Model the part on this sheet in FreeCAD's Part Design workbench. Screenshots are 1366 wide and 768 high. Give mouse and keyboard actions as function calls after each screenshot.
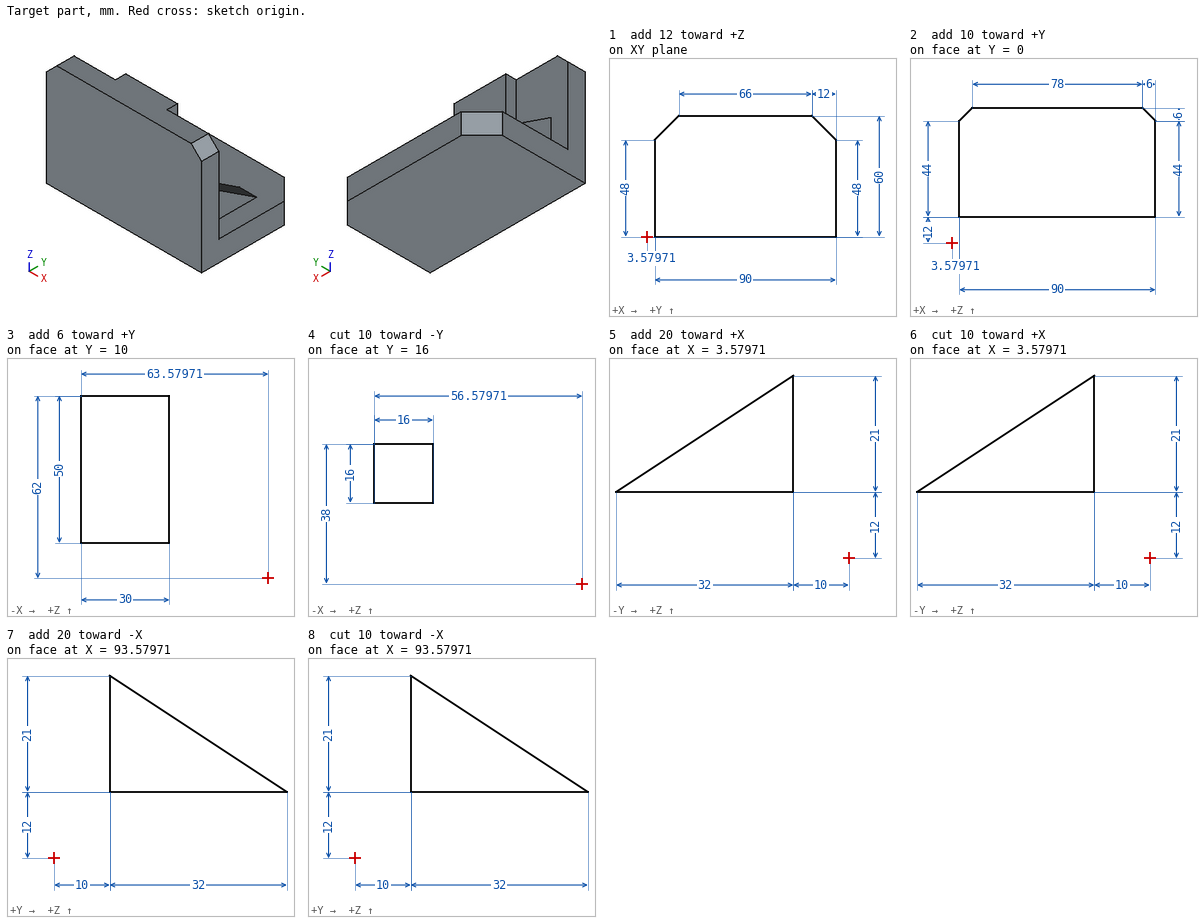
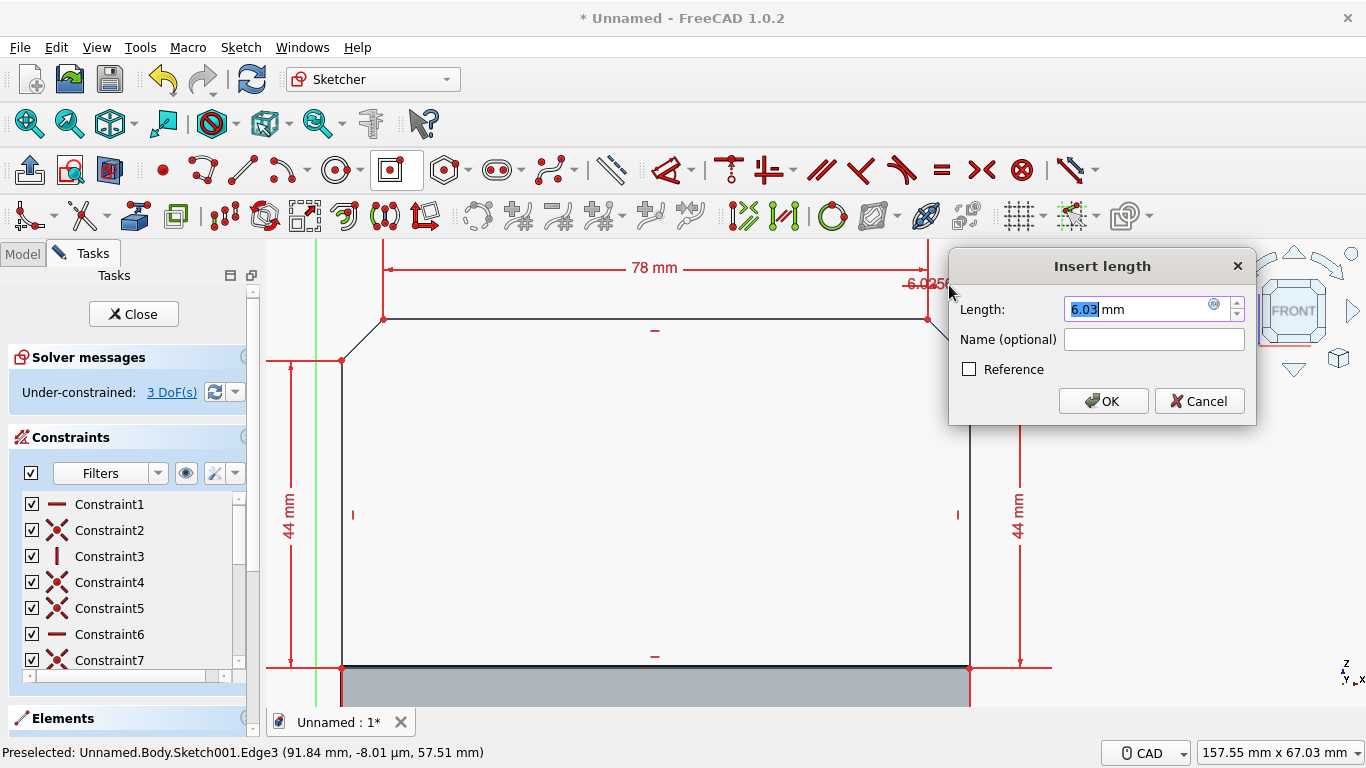
text(6)
key(Return)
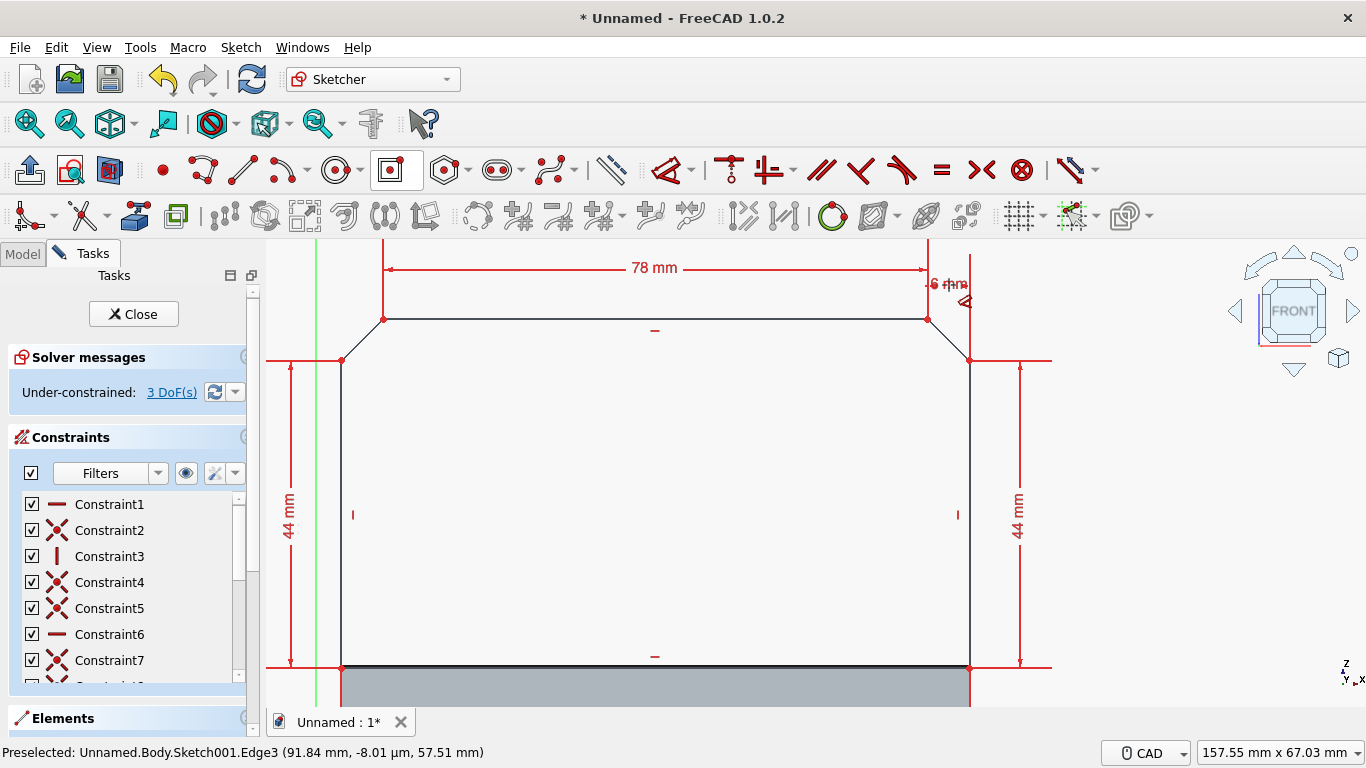
click(957, 348)
click(1004, 340)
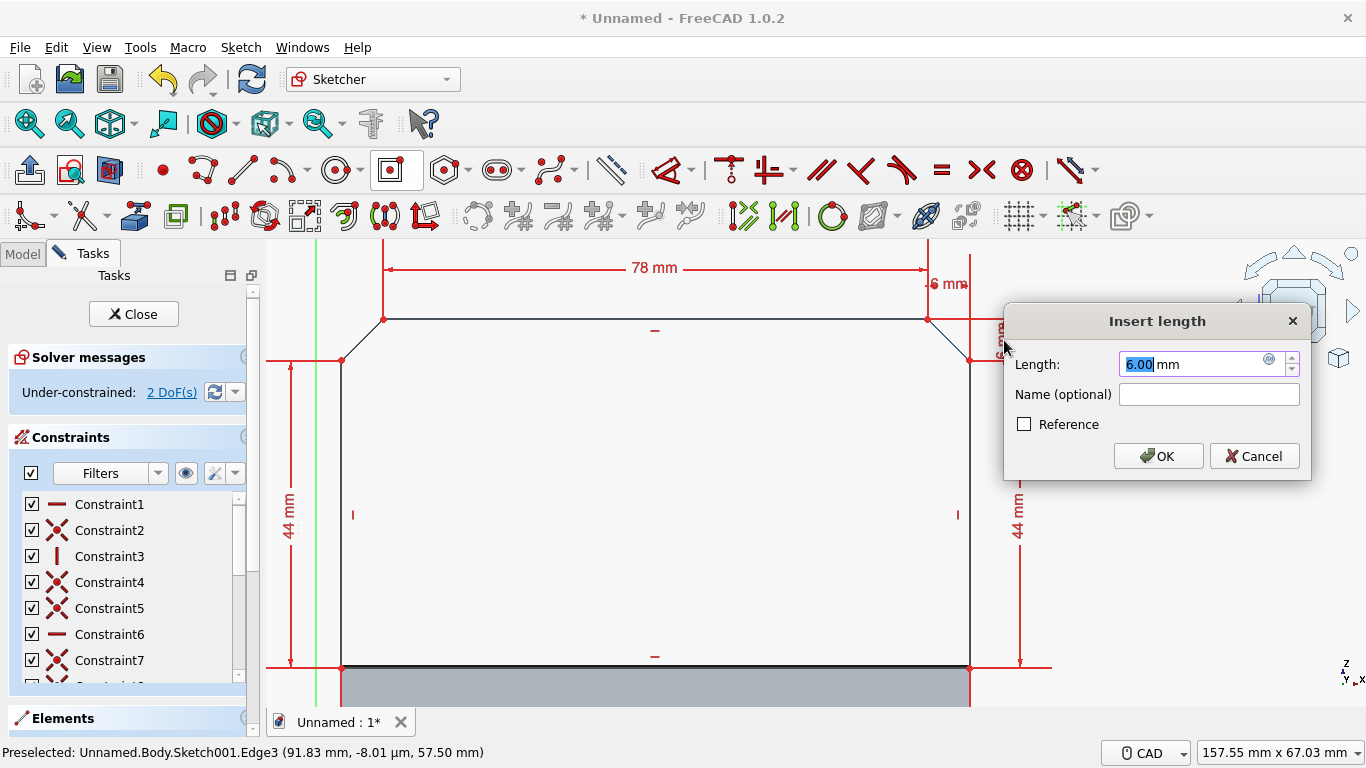
text(6)
key(Return)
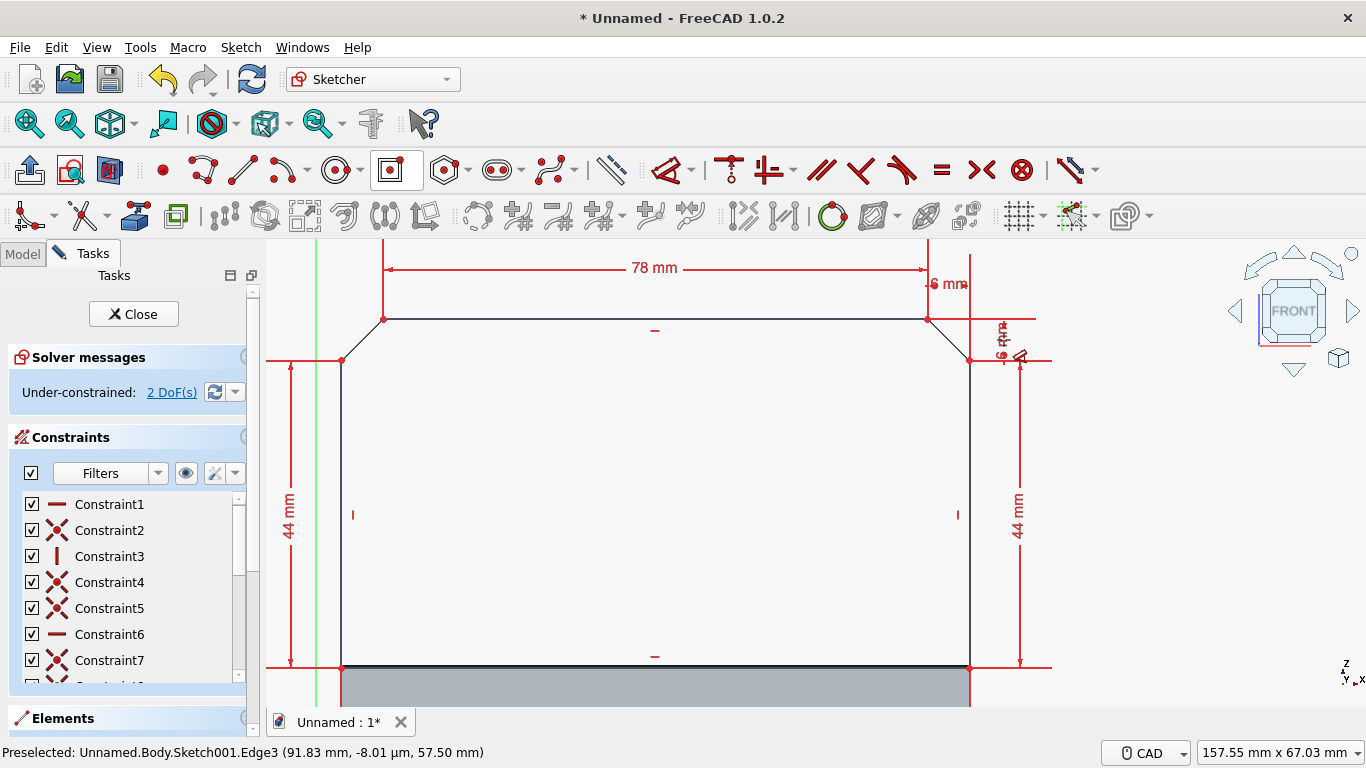
click(341, 668)
click(375, 676)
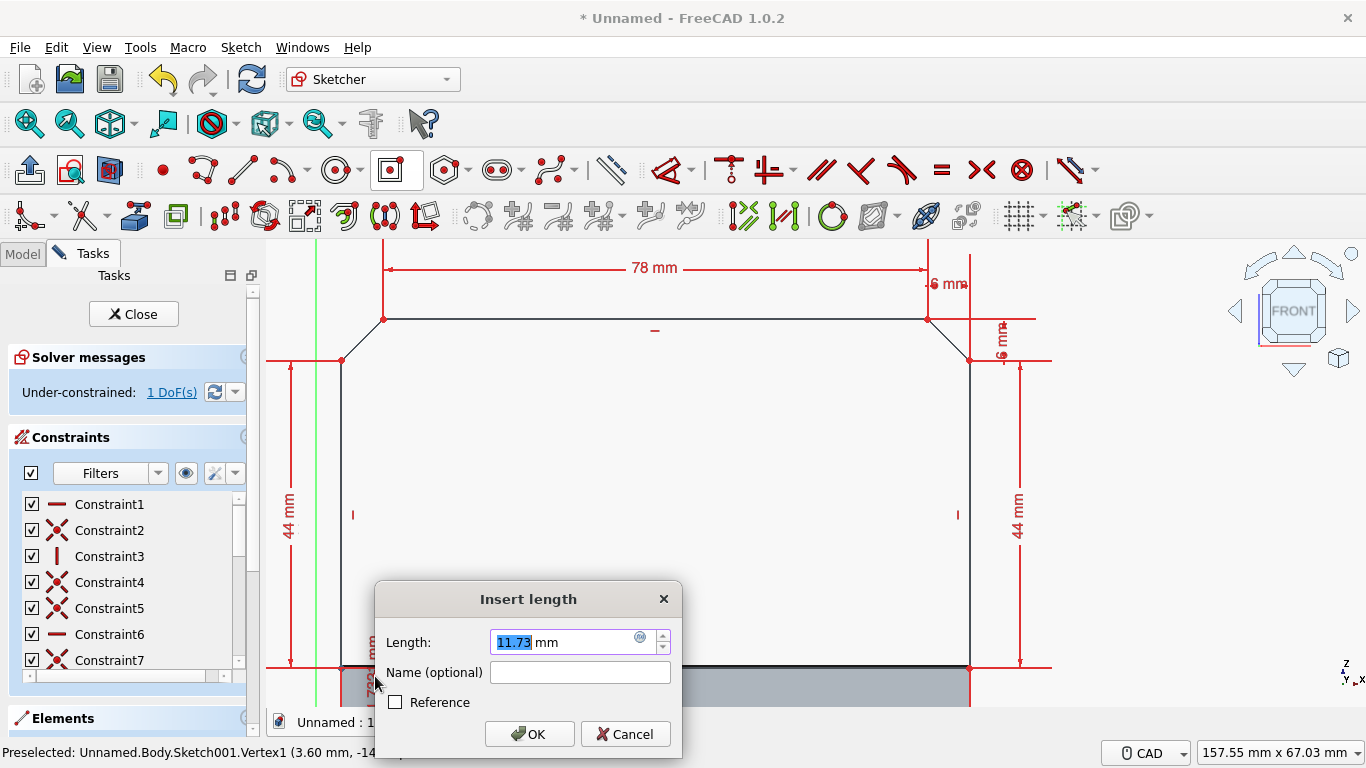
text(12)
key(Return)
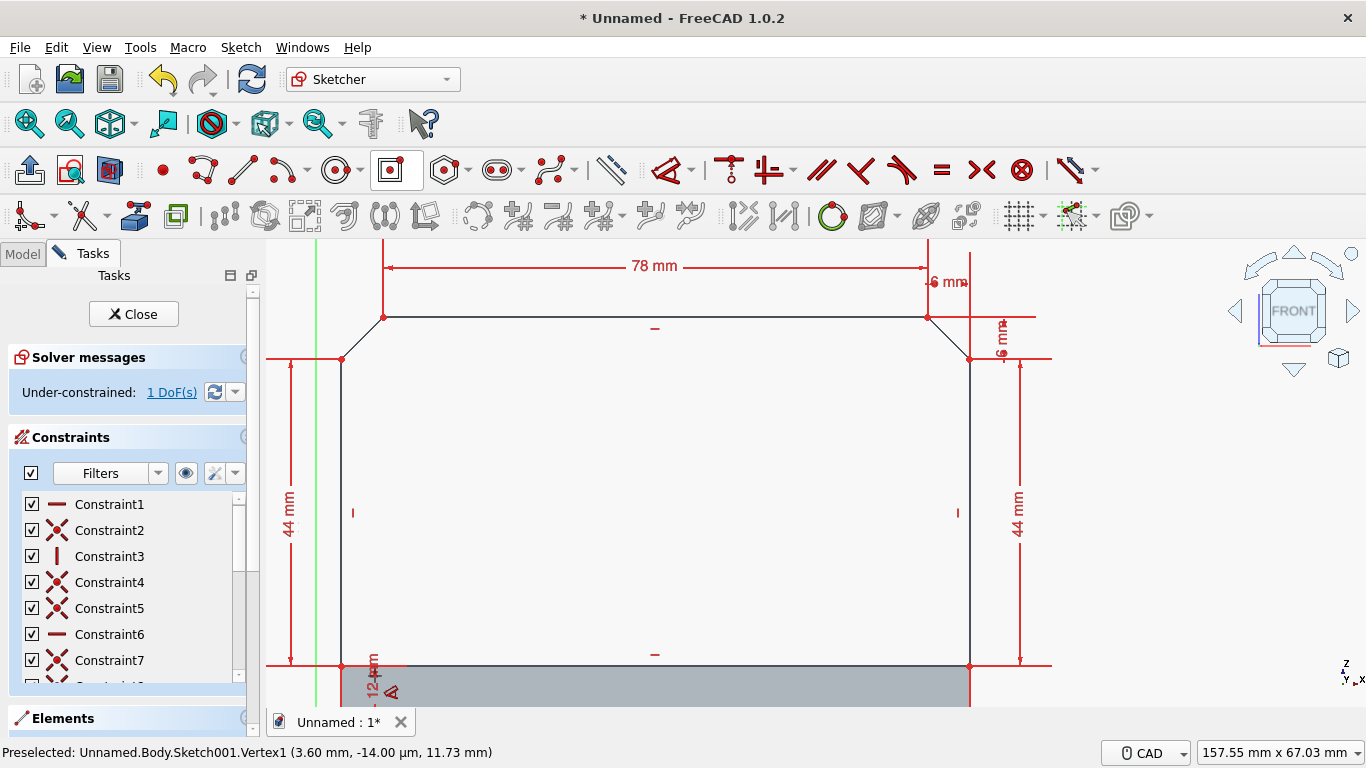
scroll(341, 666, up, 3)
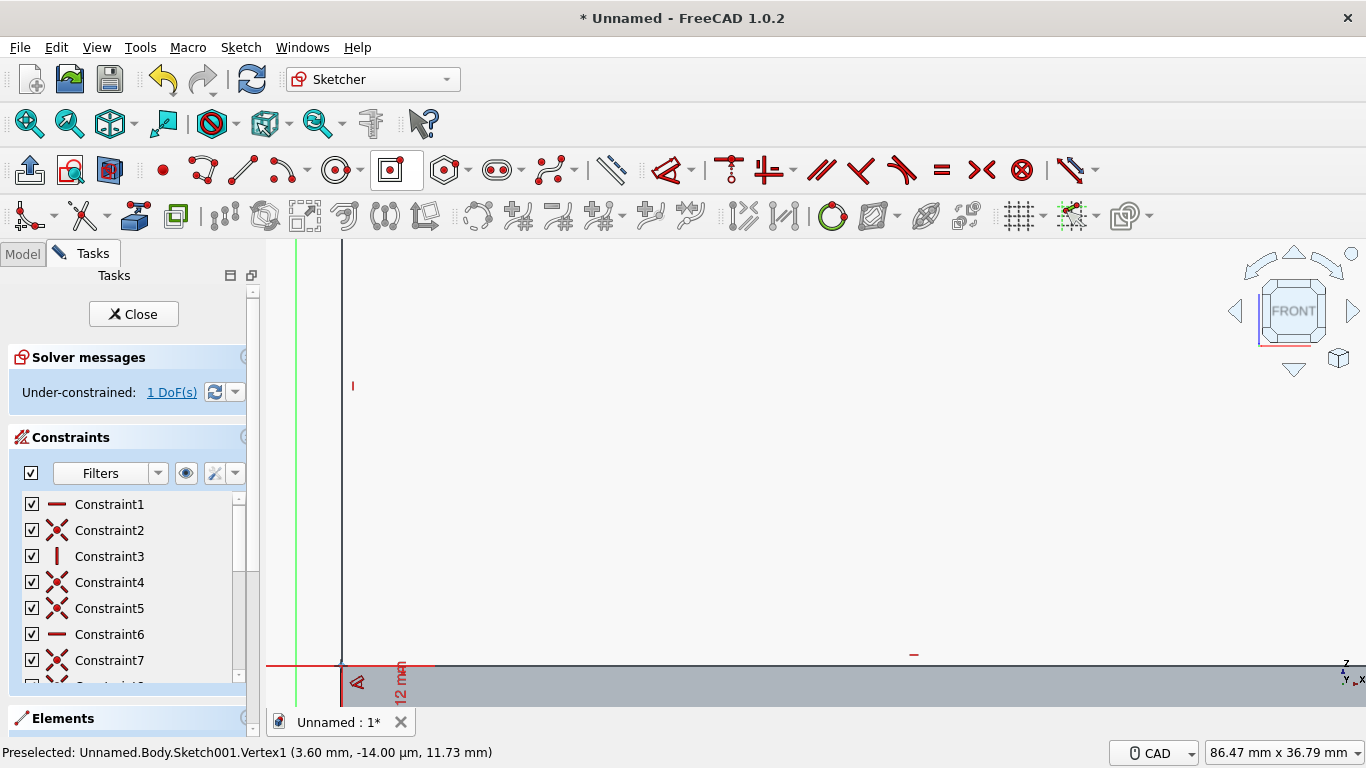
click(342, 666)
click(319, 632)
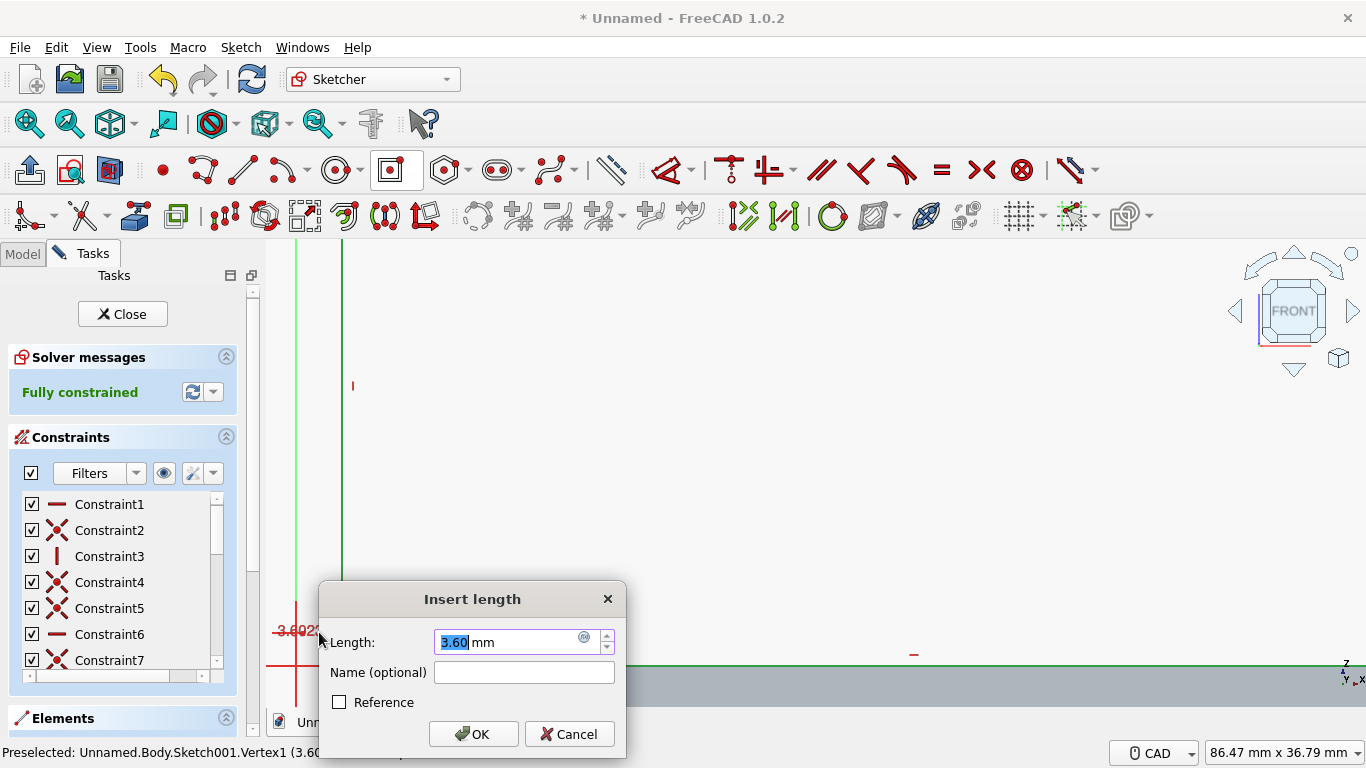
text(3.57971)
key(Return)
key(Escape)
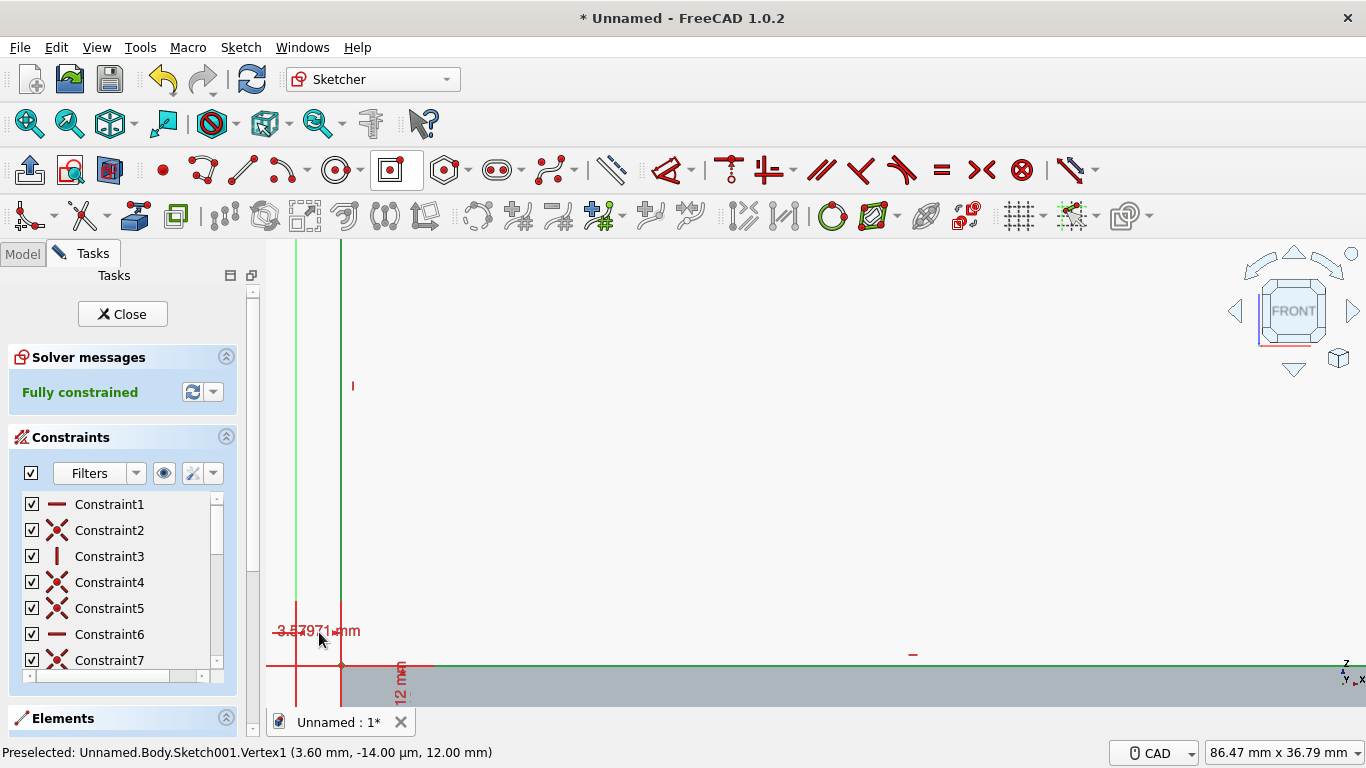
click(123, 314)